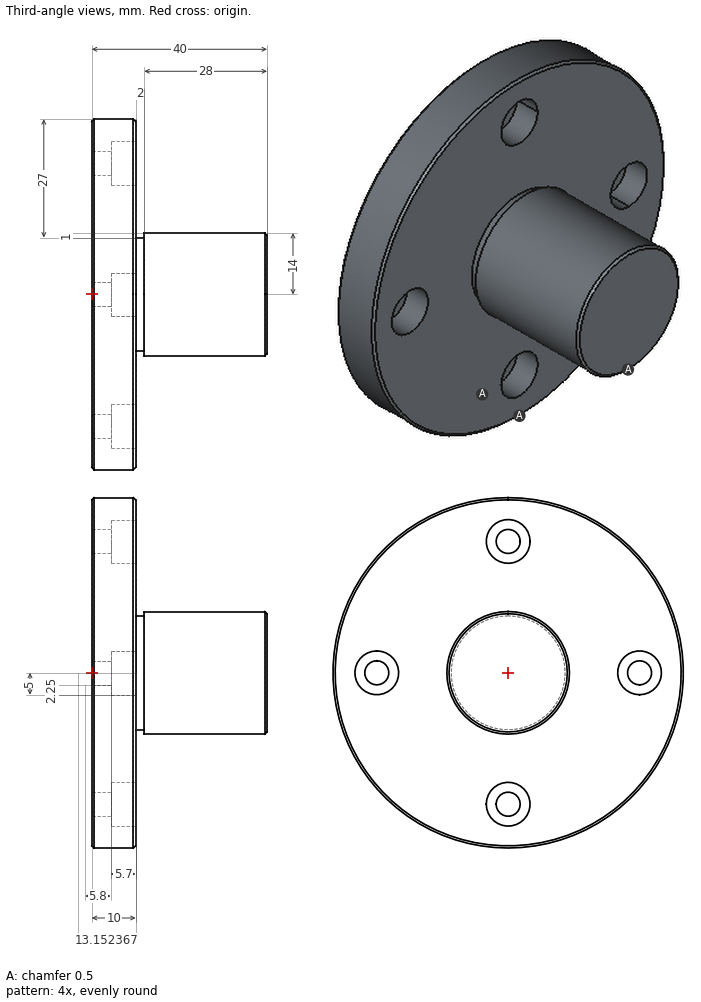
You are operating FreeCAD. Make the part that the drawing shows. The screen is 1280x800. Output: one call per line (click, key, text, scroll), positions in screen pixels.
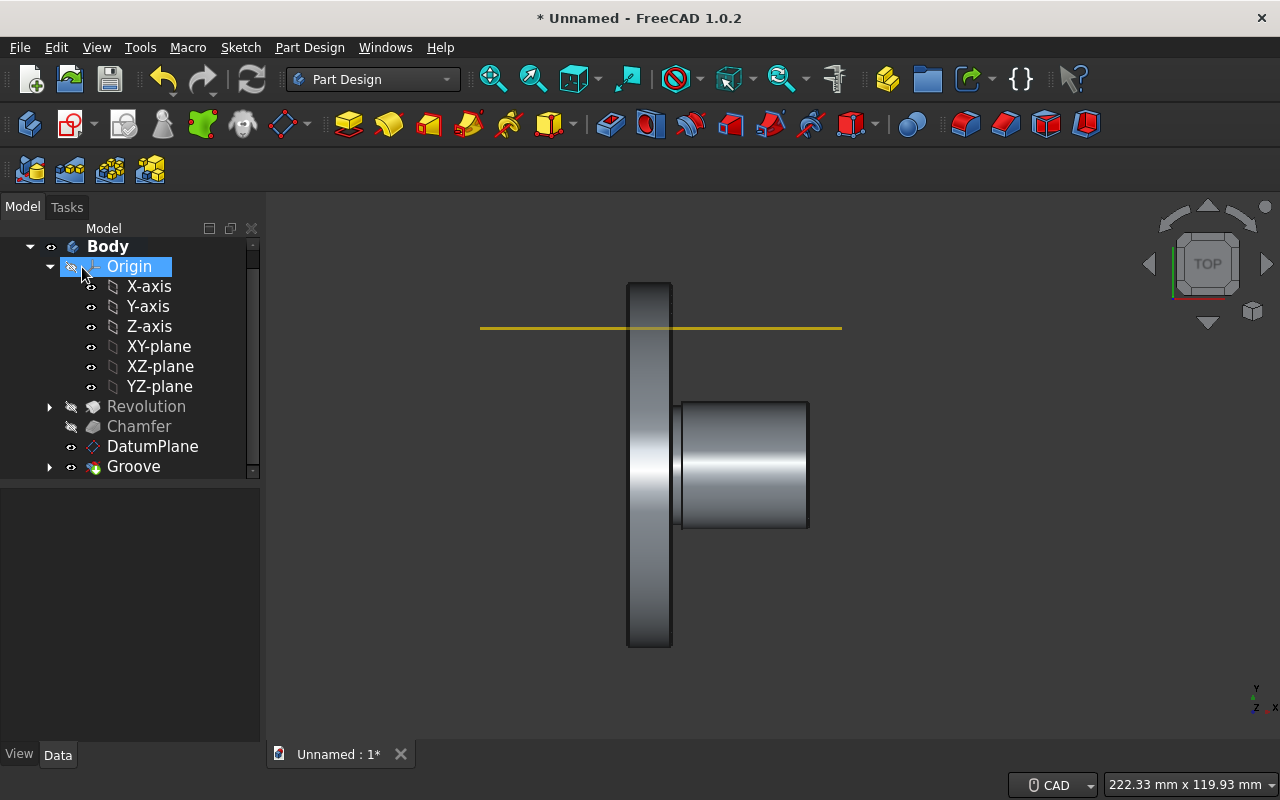
click(116, 447)
key(space)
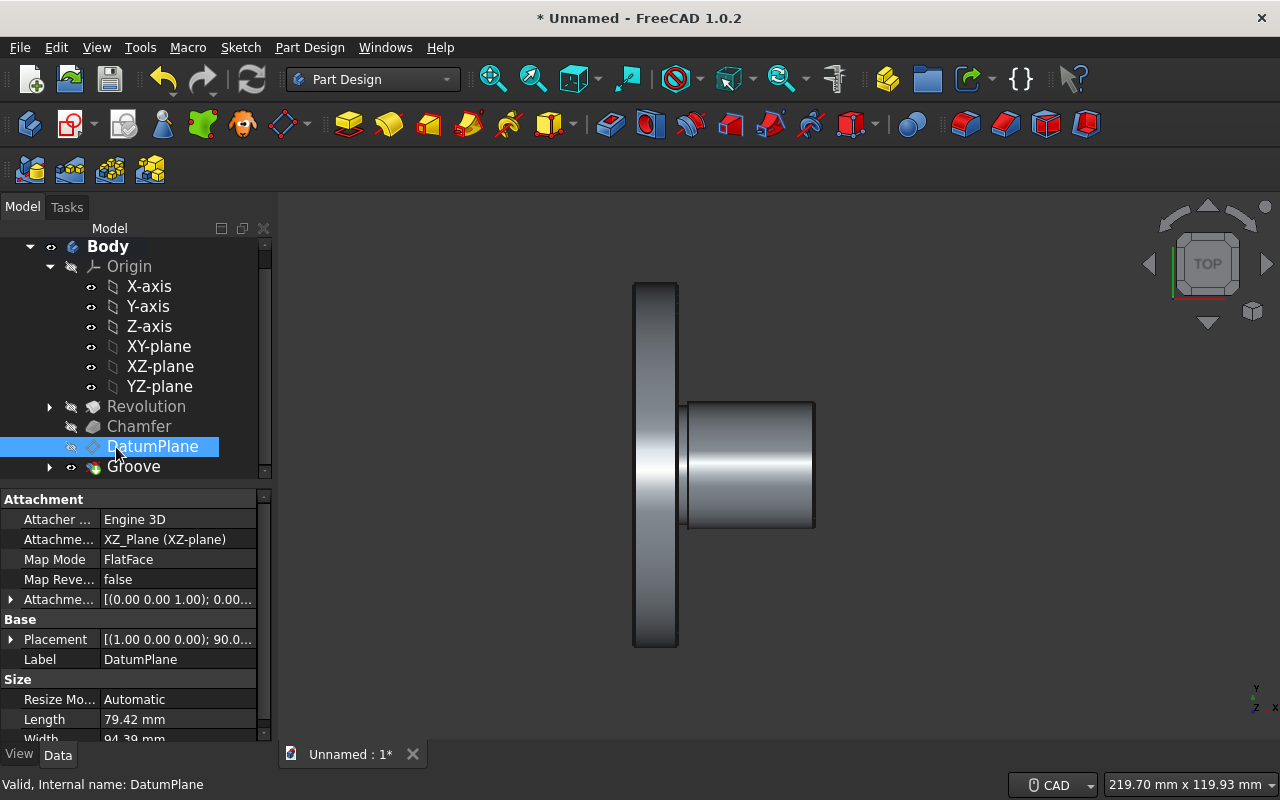
click(116, 467)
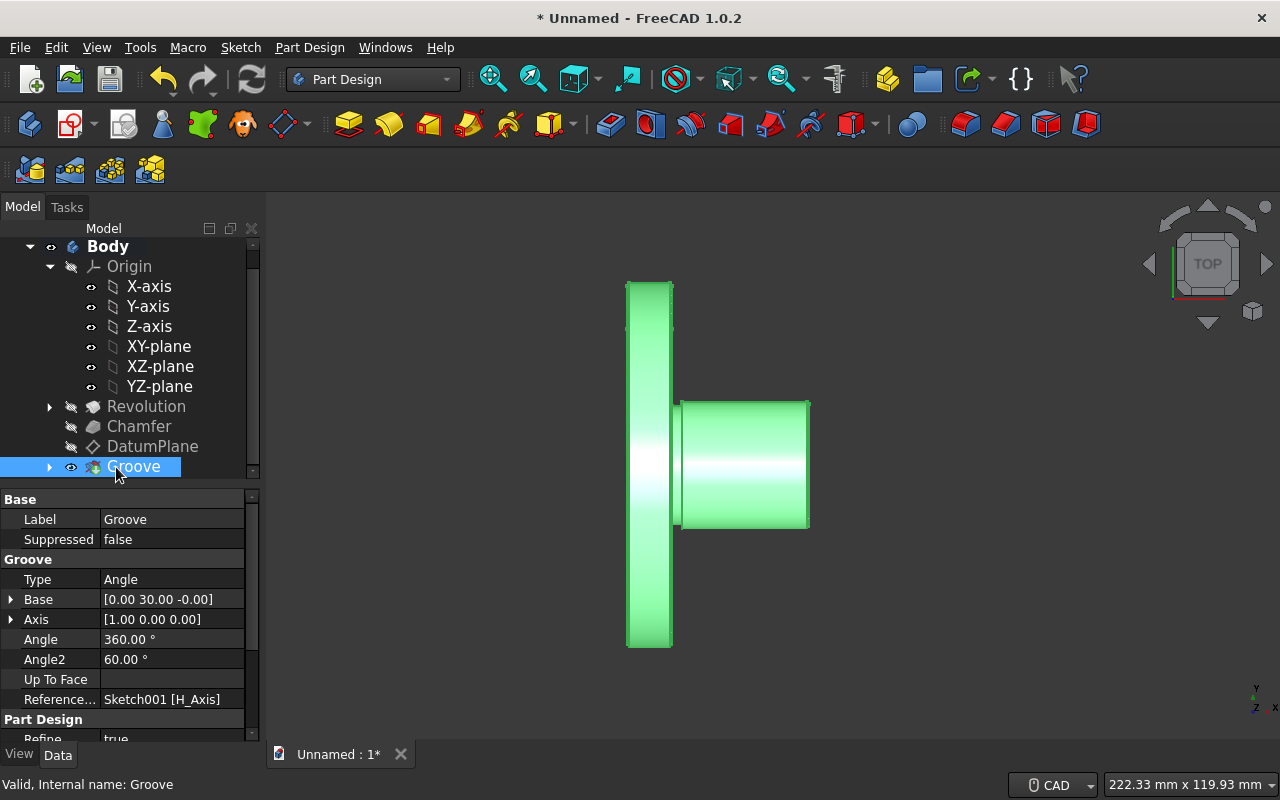
click(110, 170)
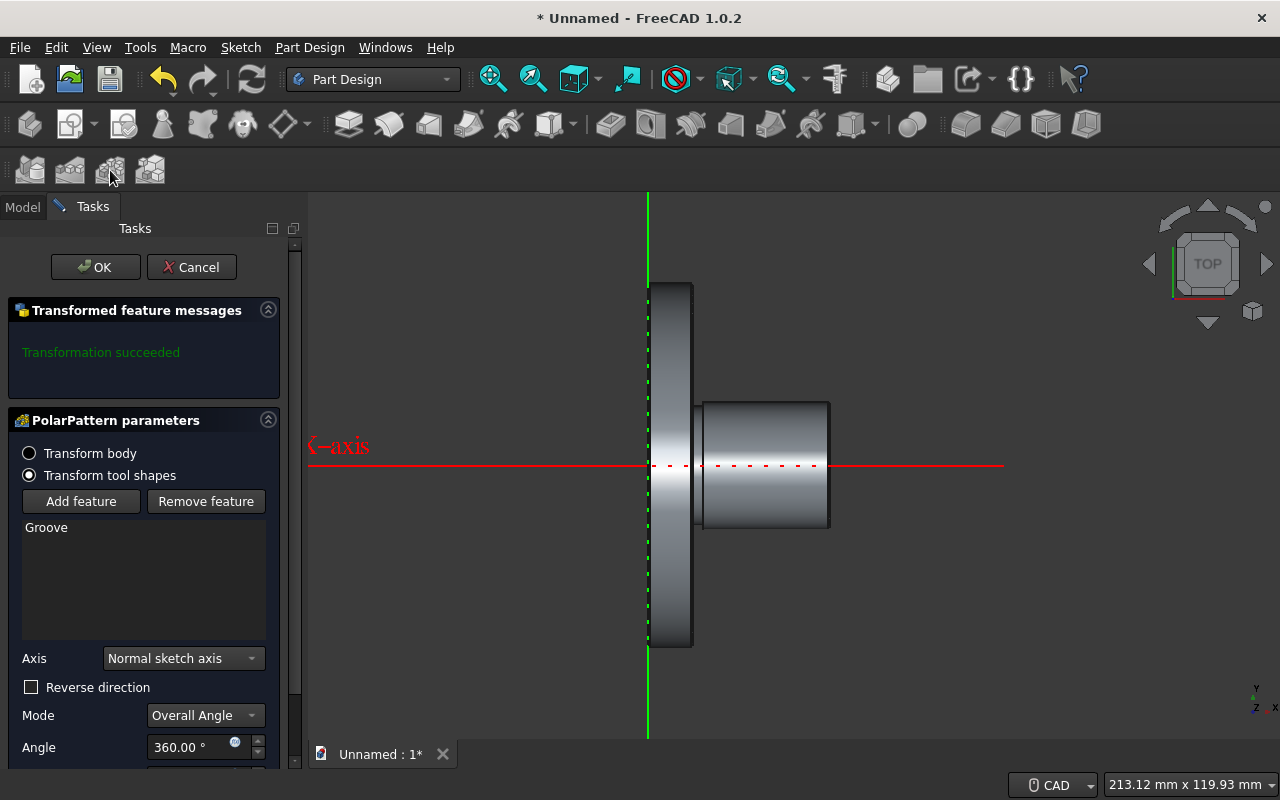
click(184, 658)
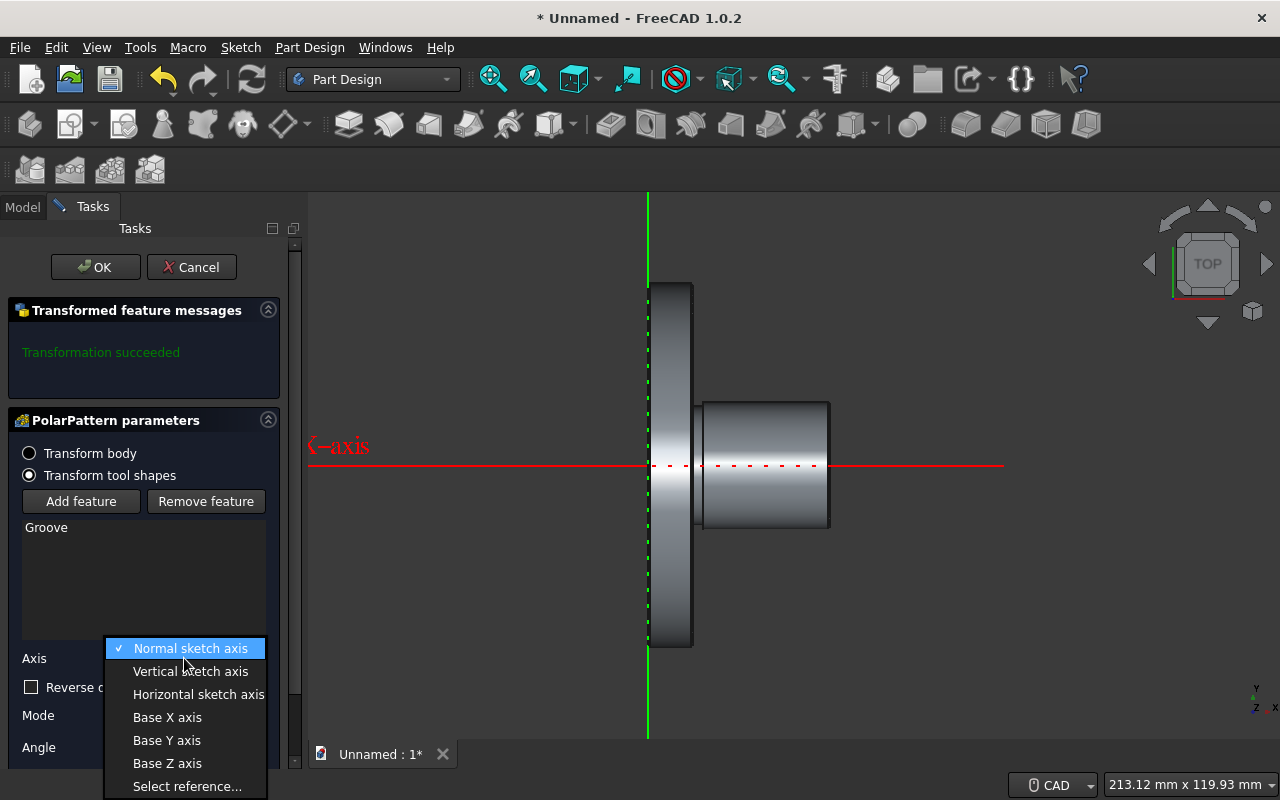
click(184, 718)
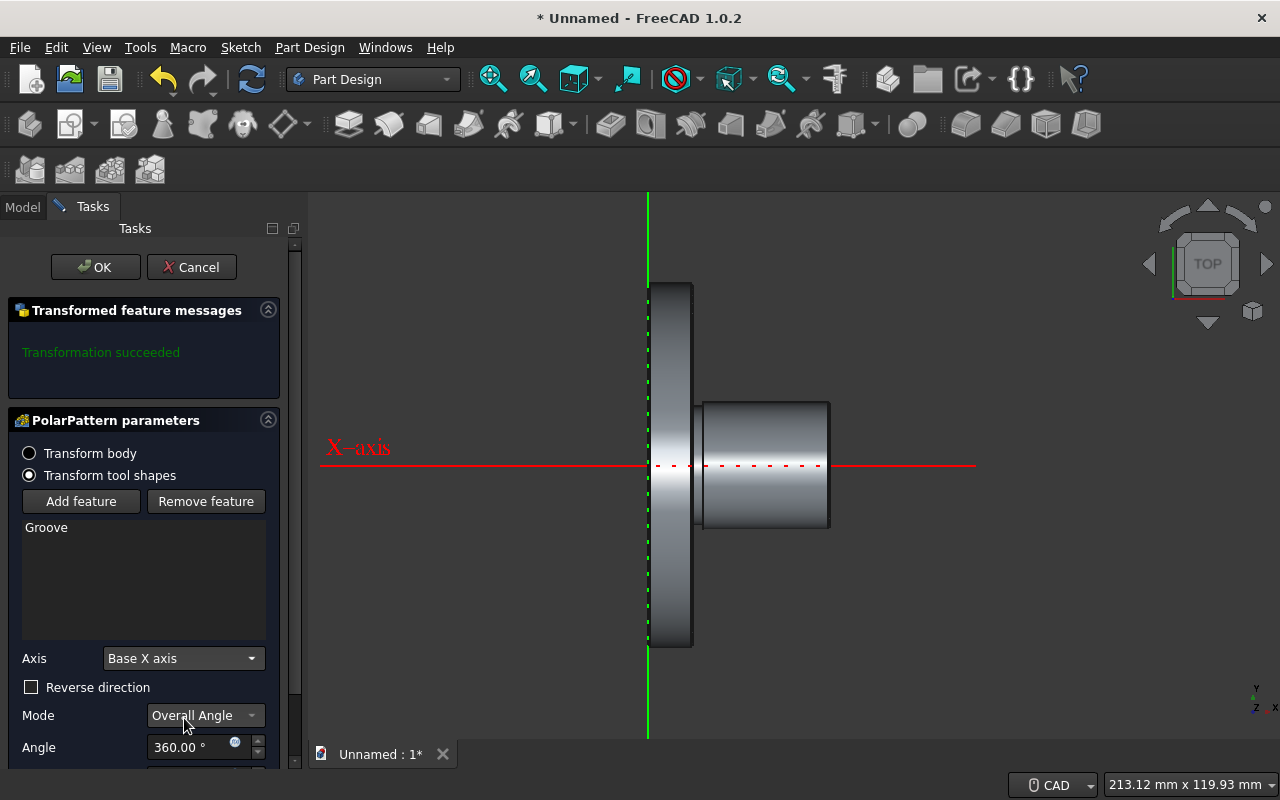
scroll(295, 503, down, 2)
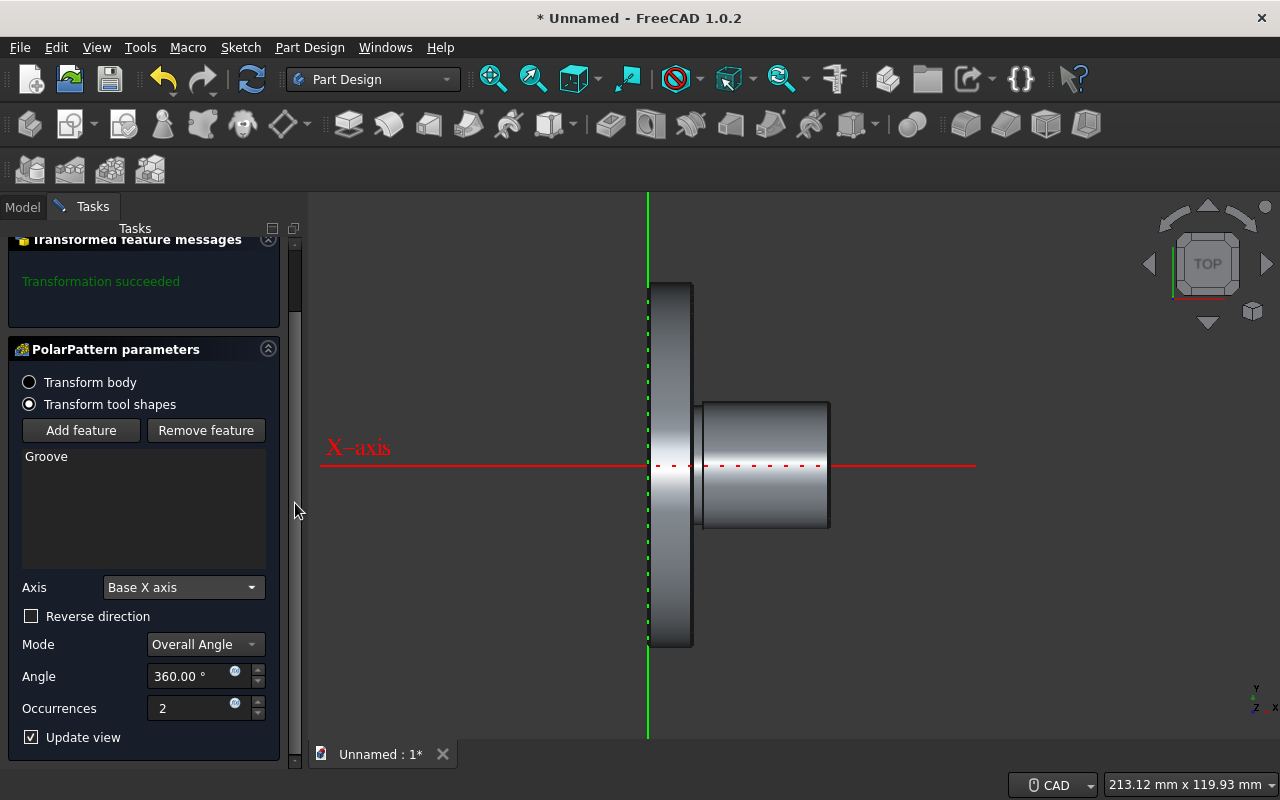
triple_click(198, 708)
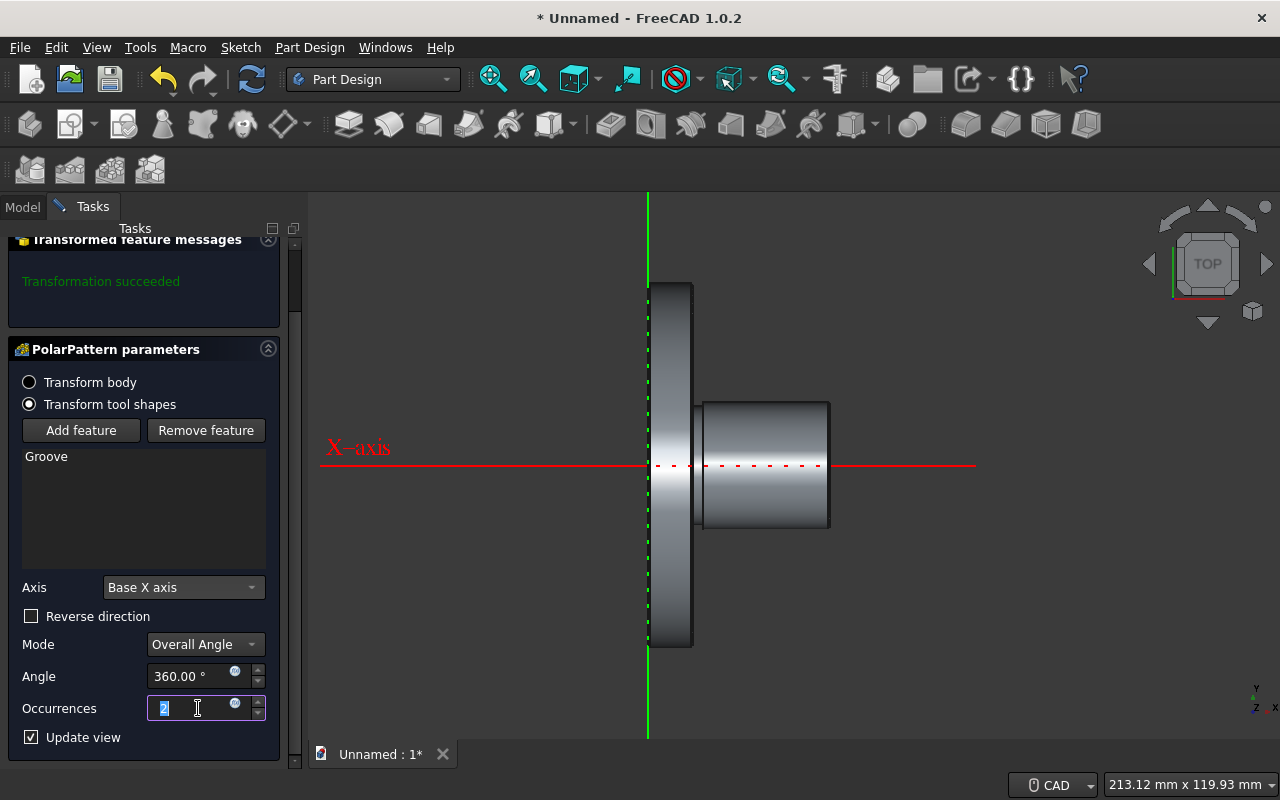
text(4)
key(Tab)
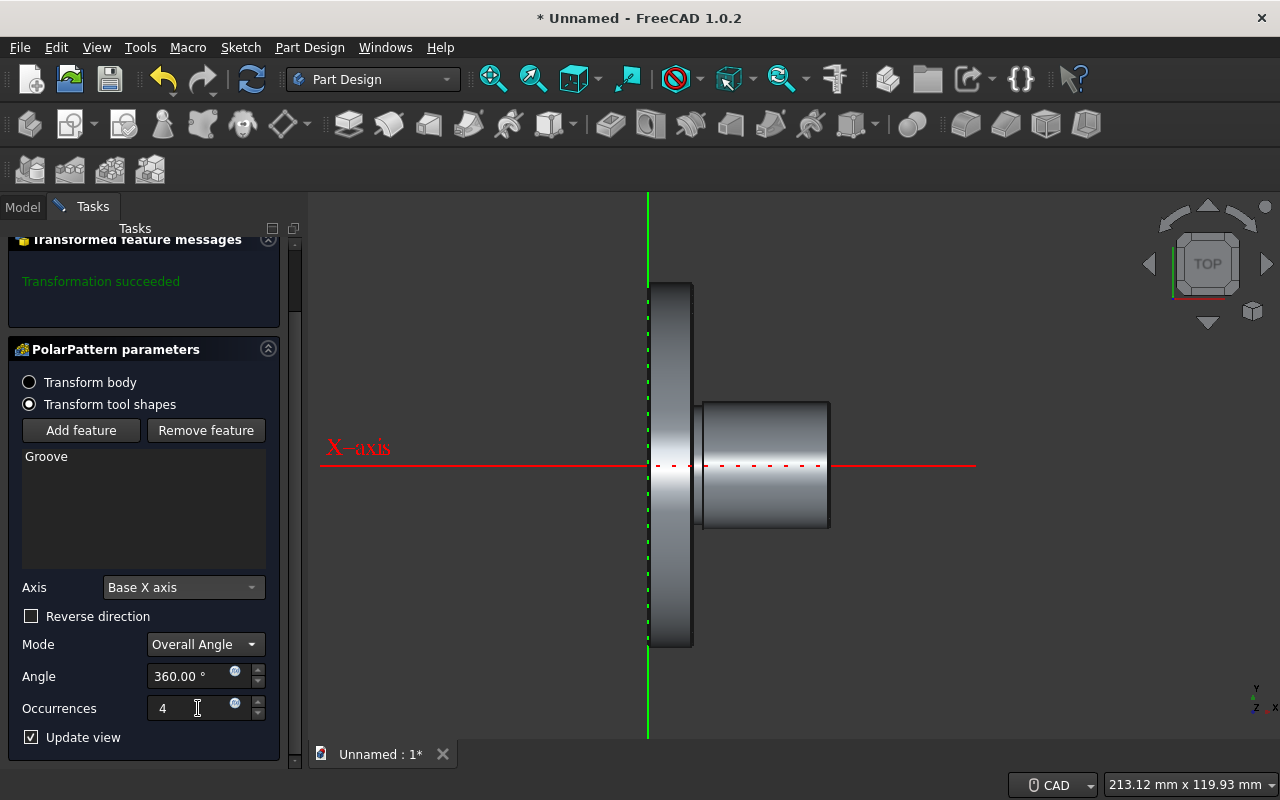
scroll(295, 503, up, 2)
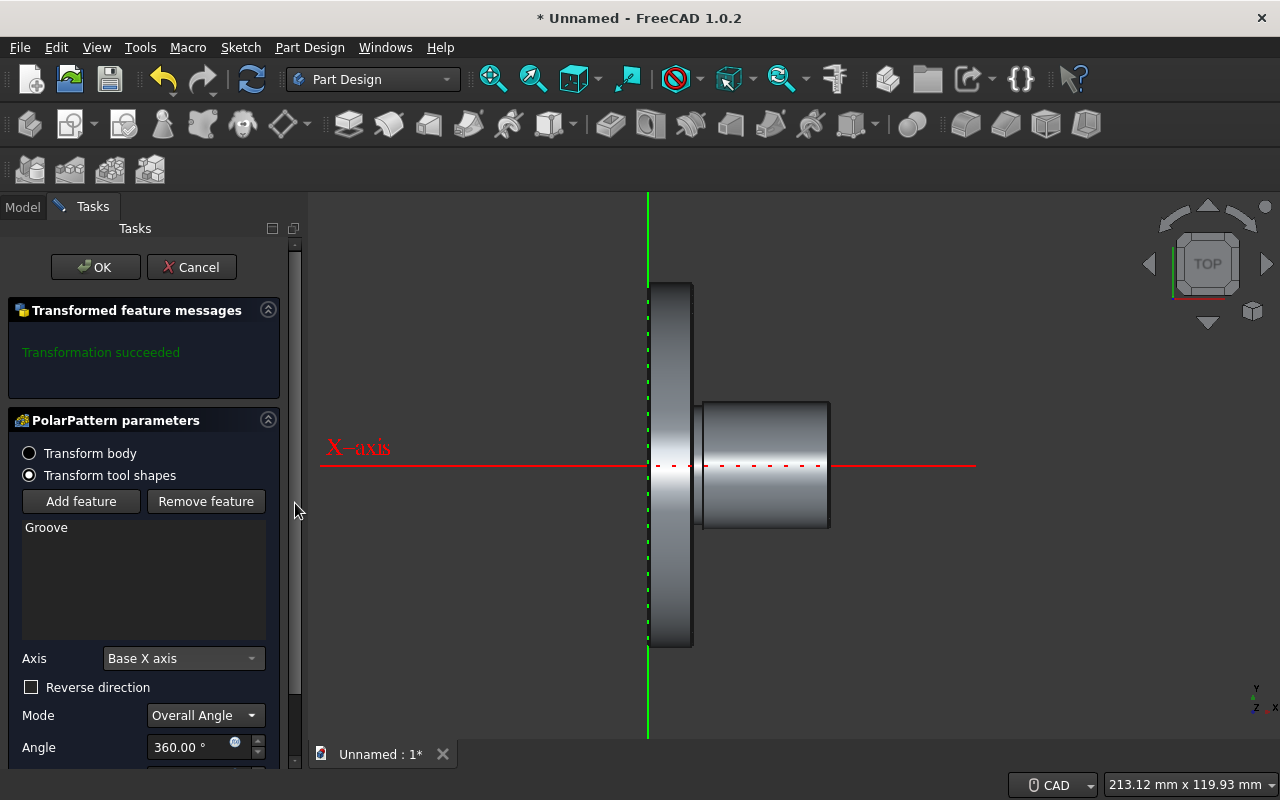
click(96, 267)